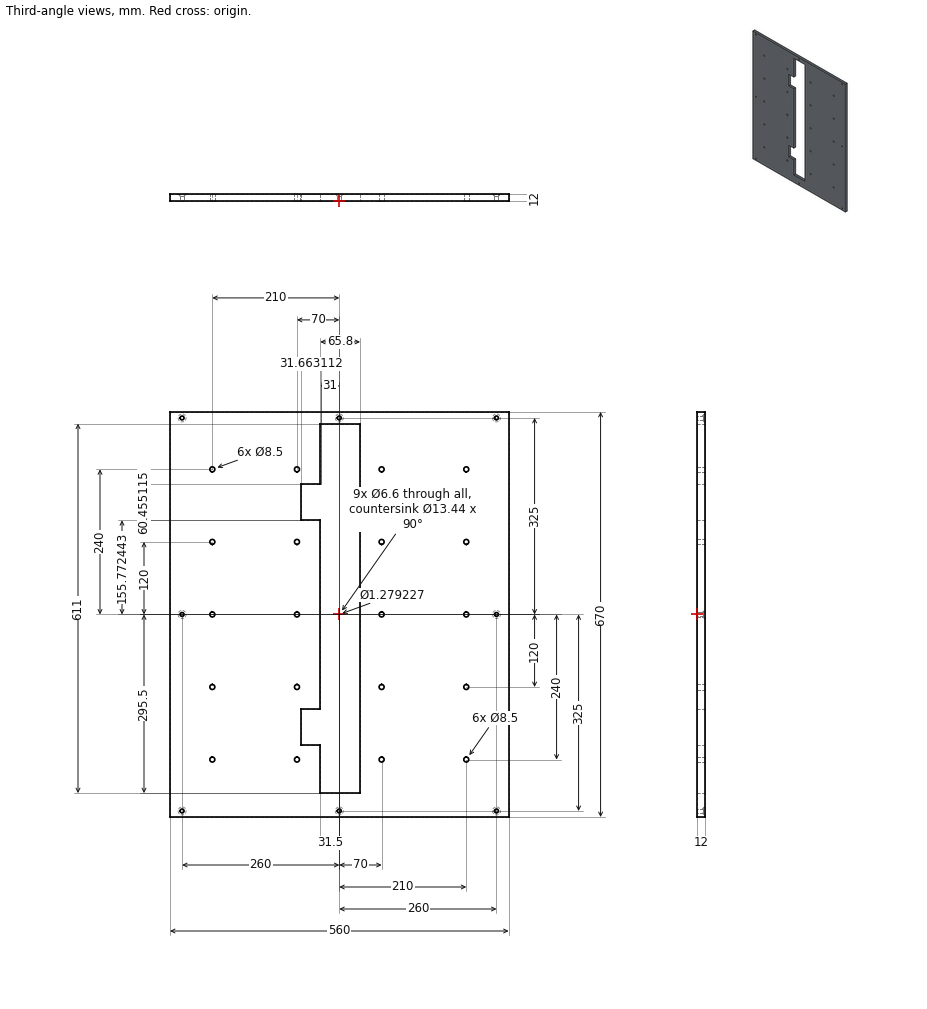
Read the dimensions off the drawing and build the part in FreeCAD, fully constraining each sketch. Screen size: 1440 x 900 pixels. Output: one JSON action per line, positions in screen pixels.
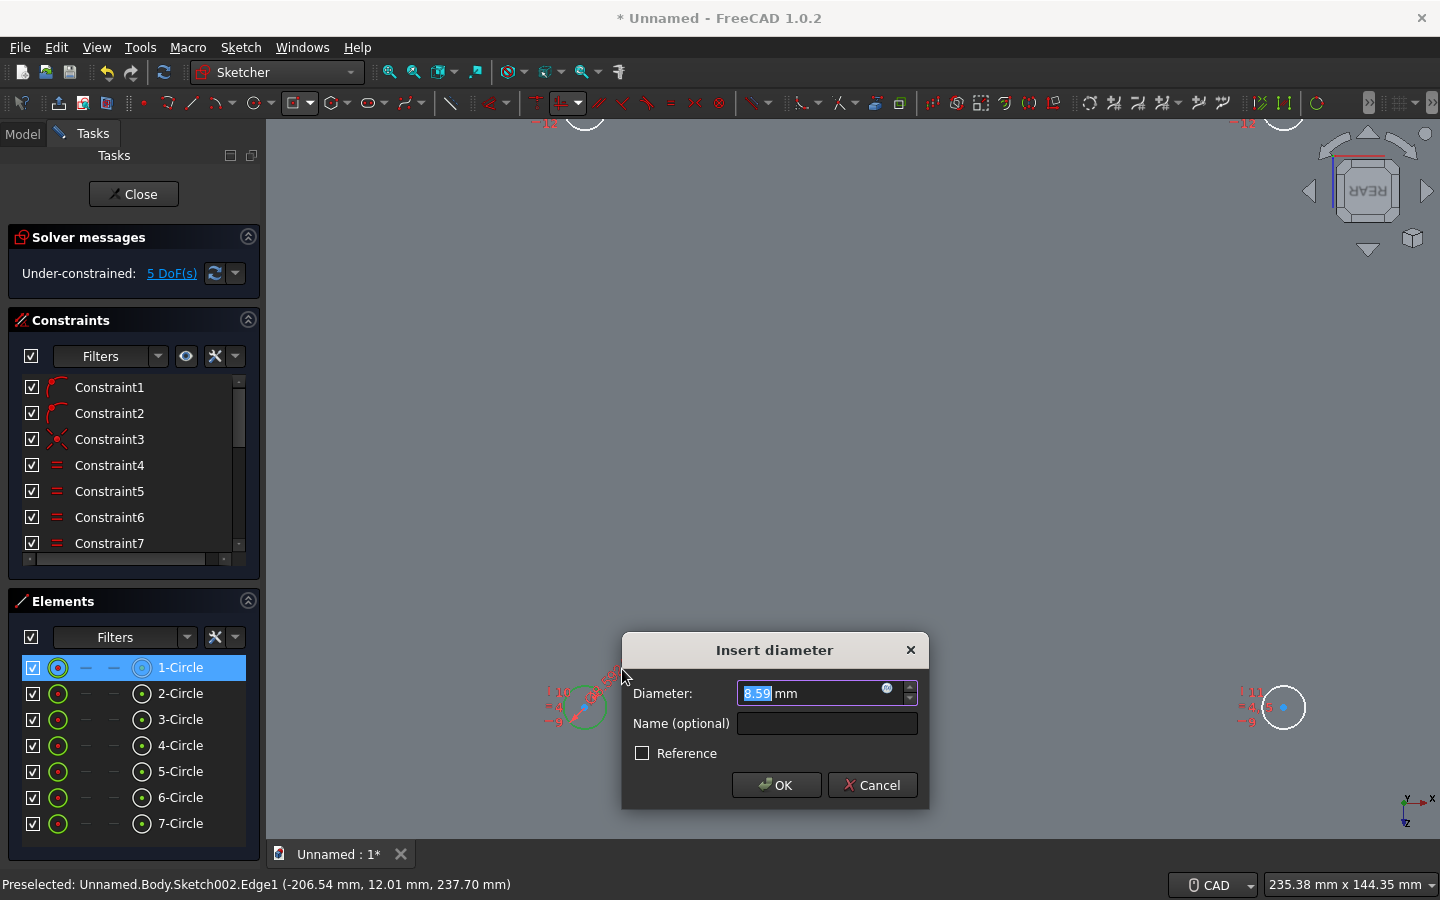
{"action": "type", "text": "8.5"}
{"action": "key", "text": "Return"}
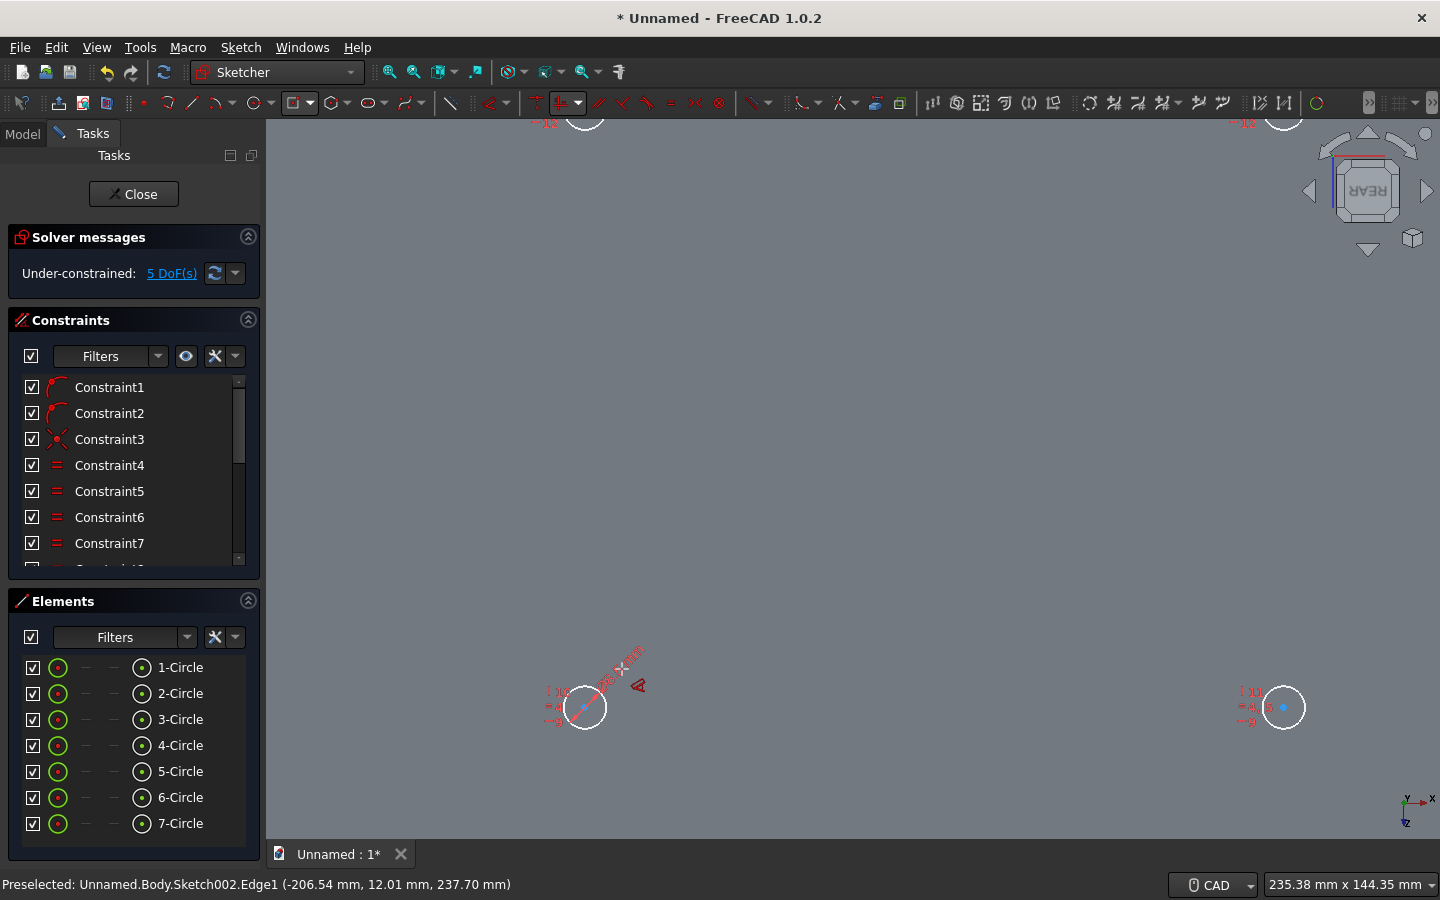
{"action": "scroll", "coordinate": [601, 695], "scroll_direction": "down", "scroll_amount": 5}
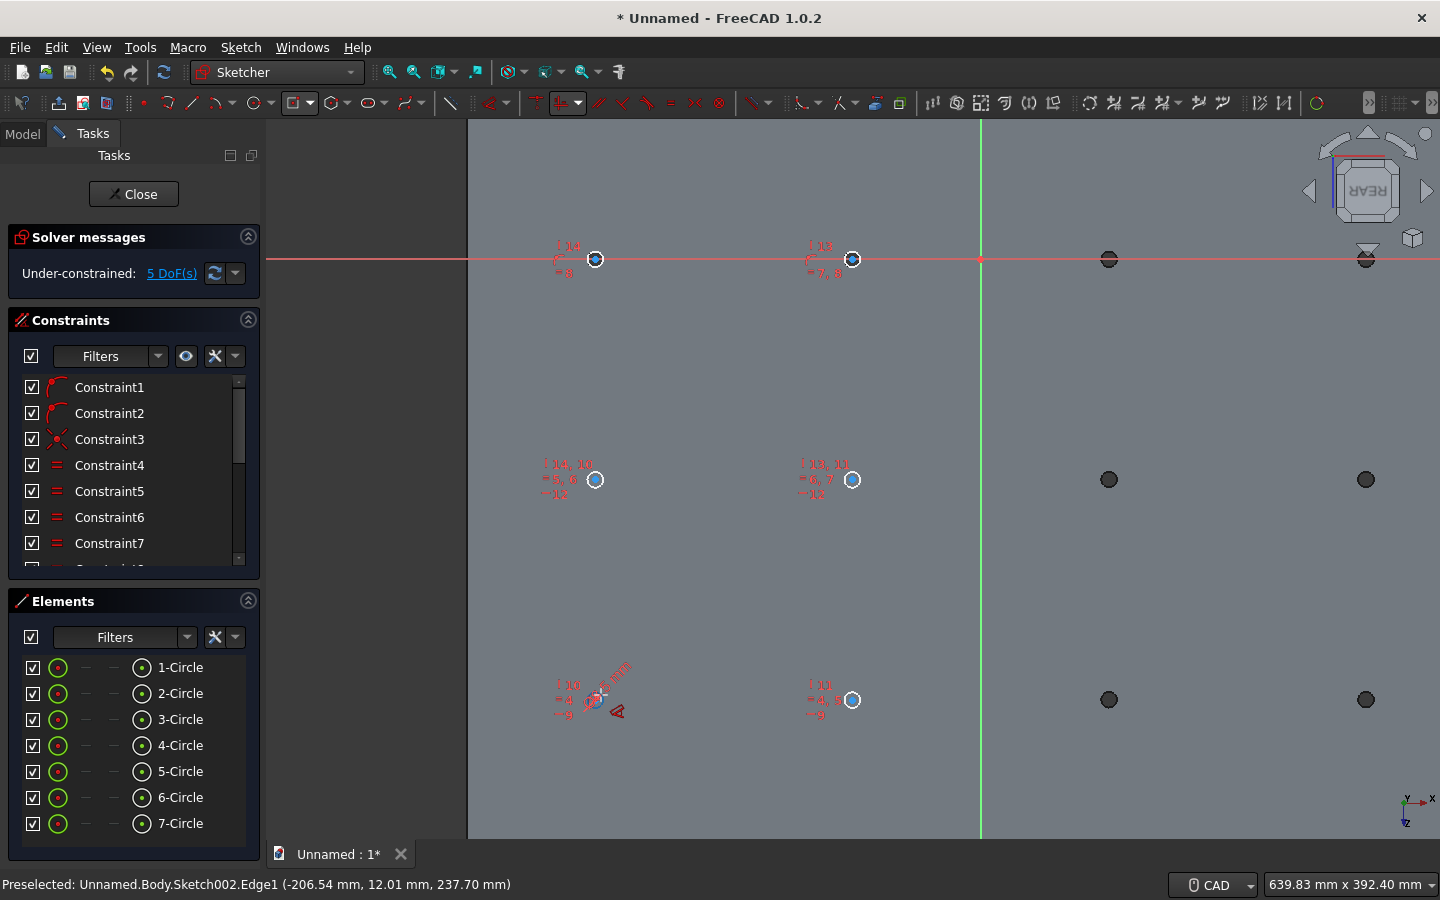
{"action": "scroll", "coordinate": [981, 259], "scroll_direction": "up", "scroll_amount": 15}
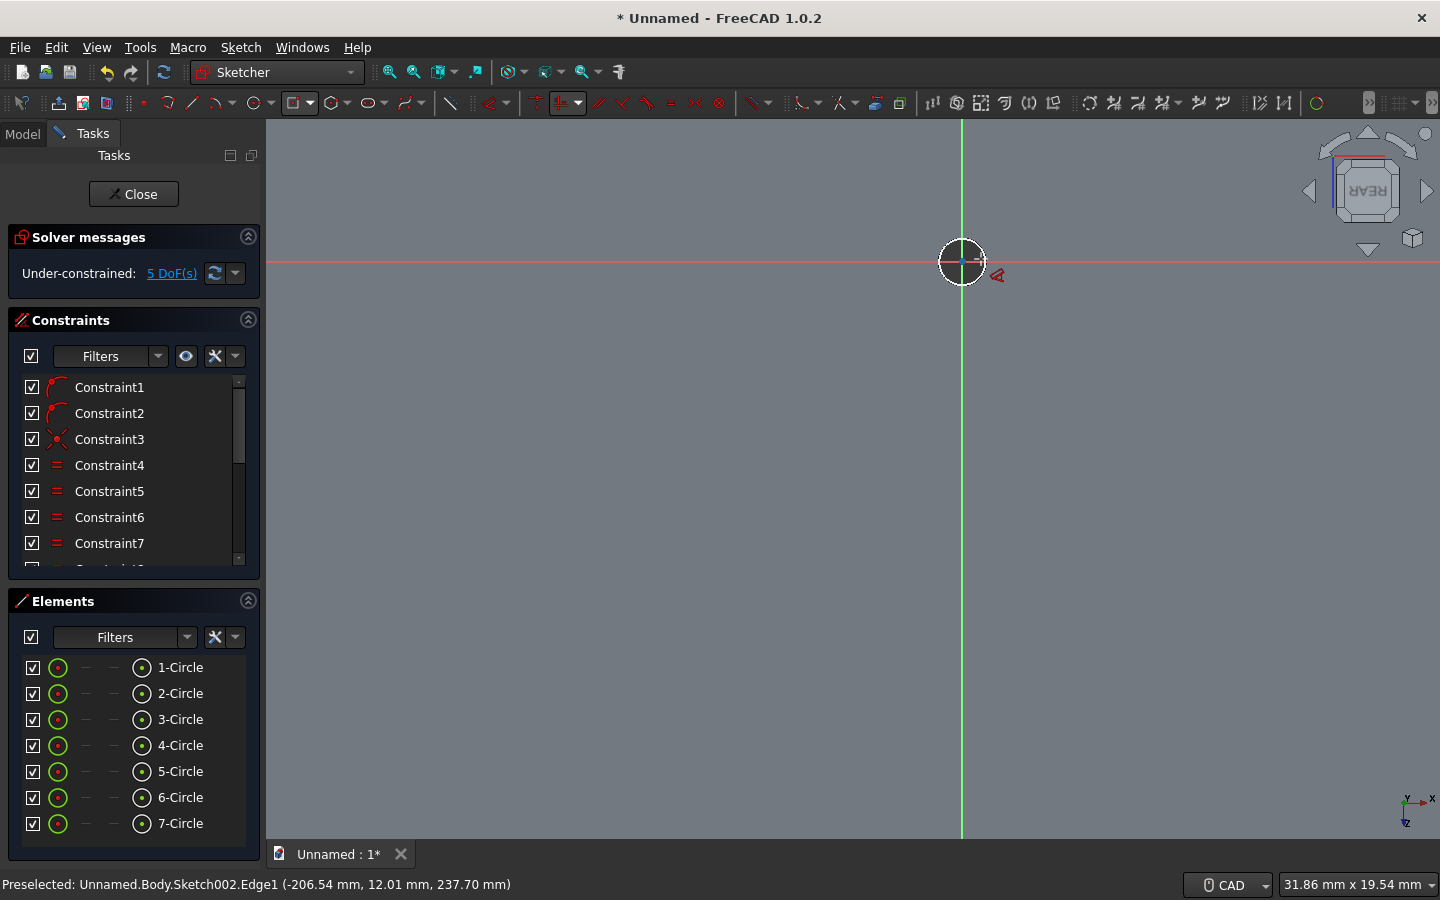
{"action": "left_click", "coordinate": [979, 246]}
{"action": "left_click", "coordinate": [1002, 224]}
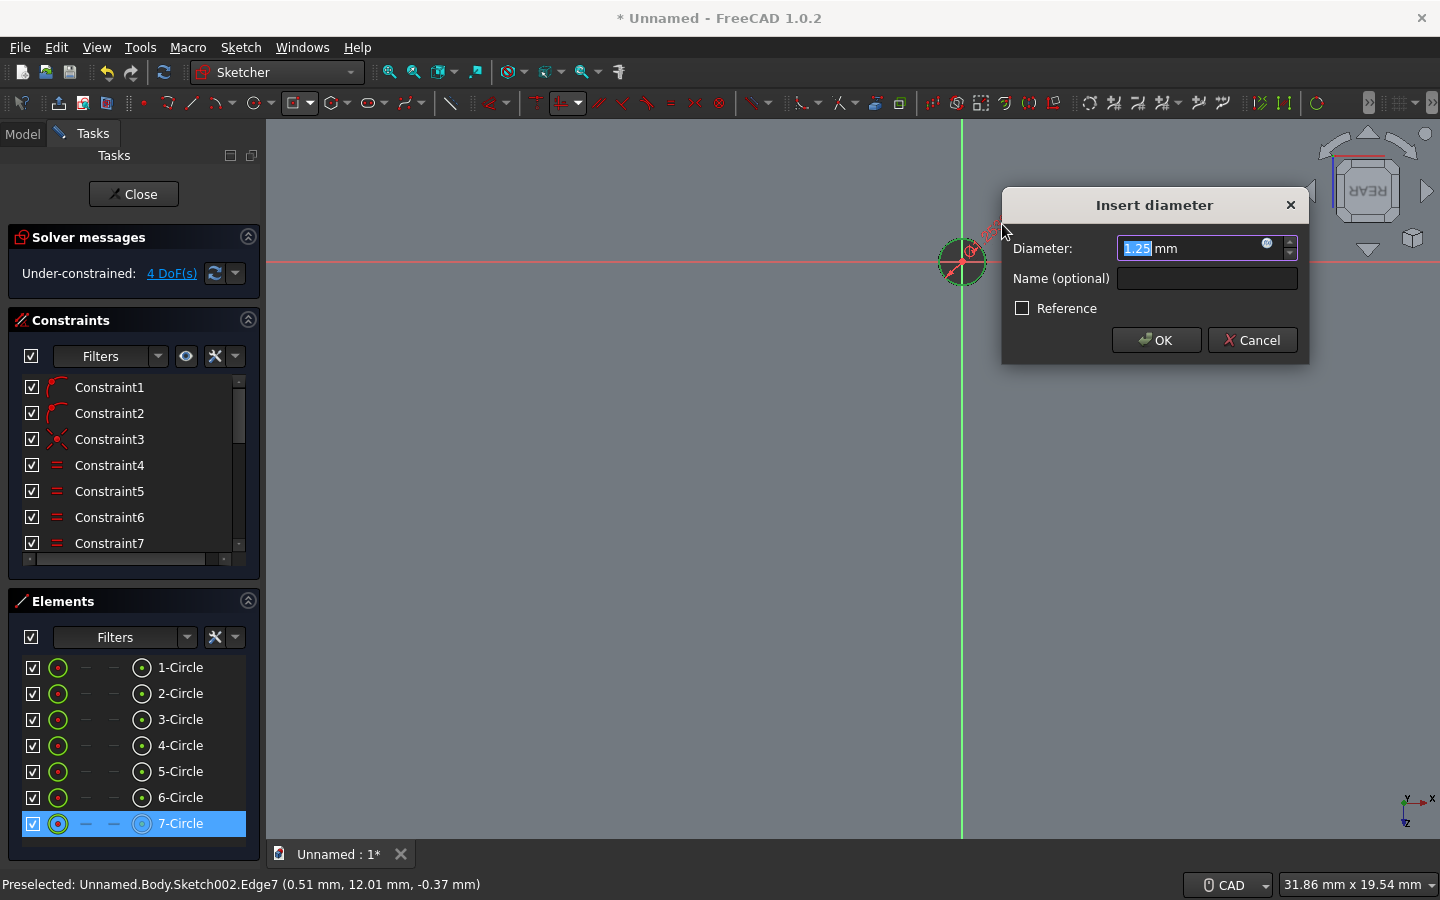
{"action": "type", "text": "1.279227"}
{"action": "key", "text": "Return"}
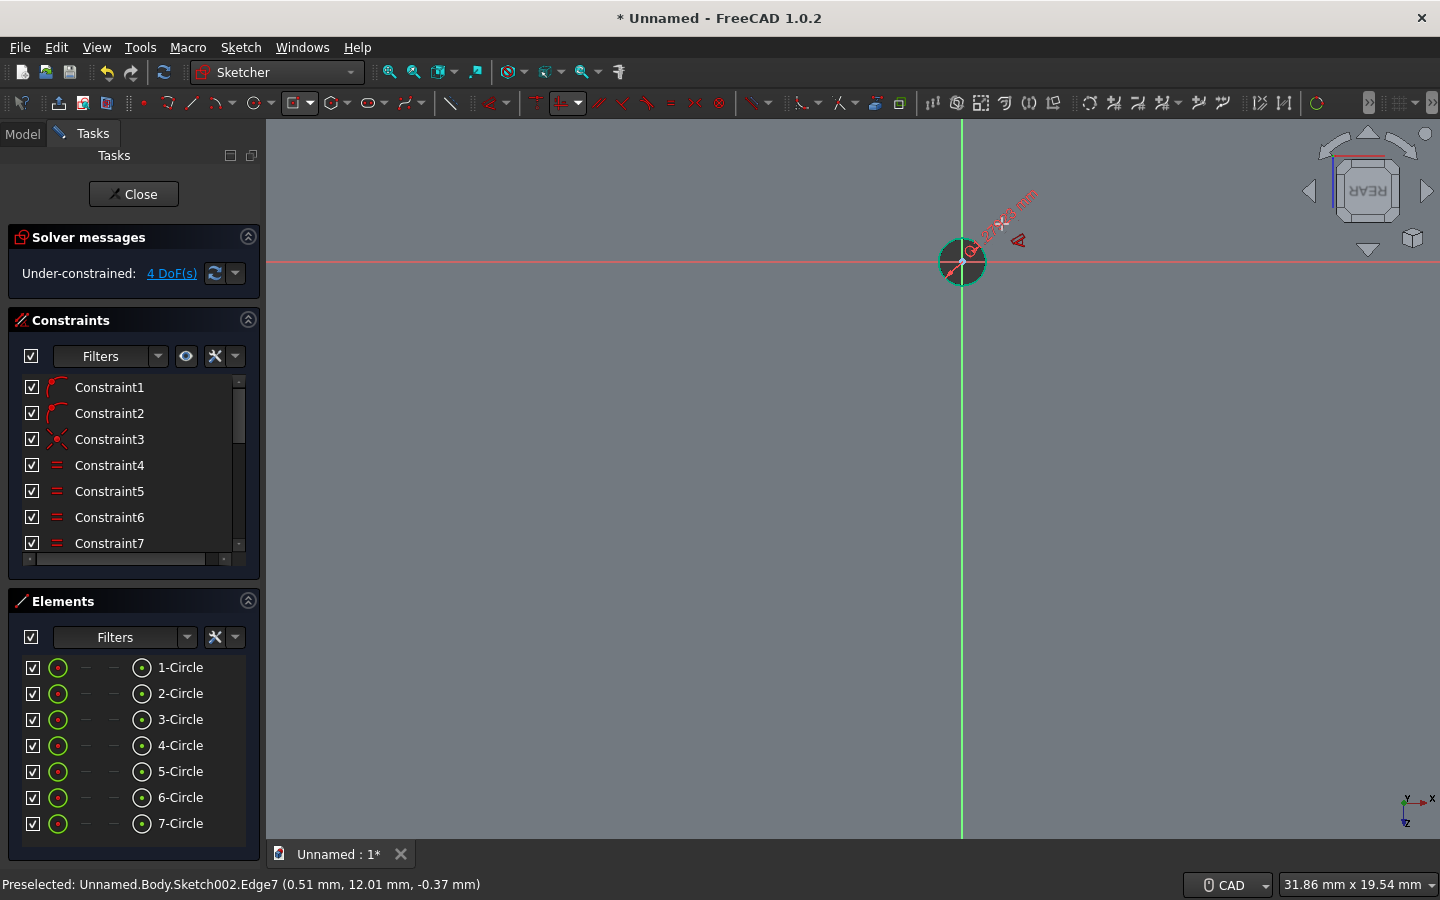
{"action": "scroll", "coordinate": [981, 259], "scroll_direction": "down", "scroll_amount": 15}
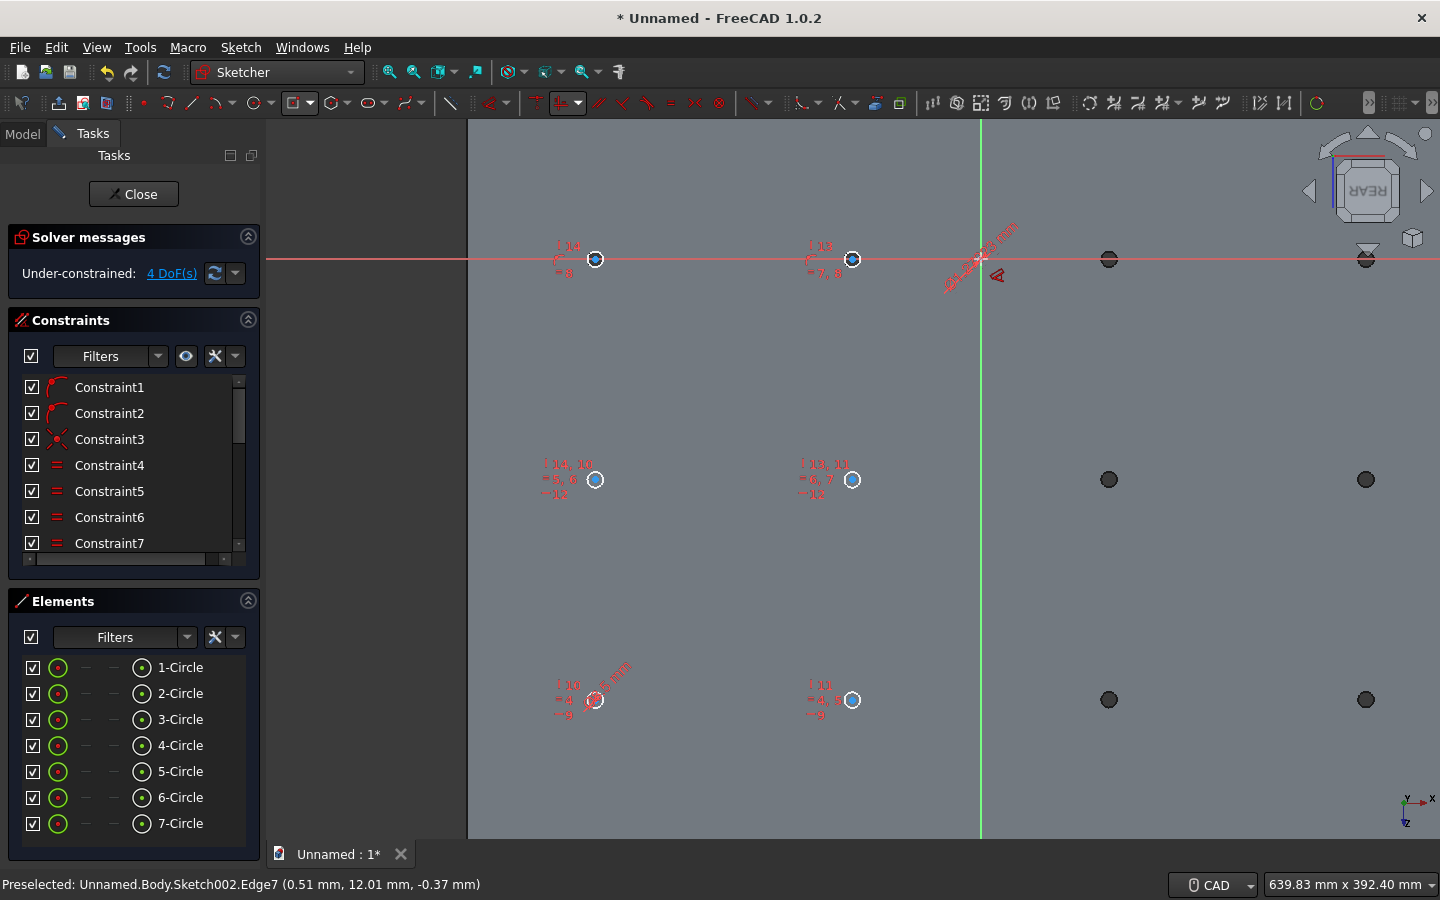
{"action": "left_click", "coordinate": [852, 700]}
{"action": "left_click", "coordinate": [916, 734]}